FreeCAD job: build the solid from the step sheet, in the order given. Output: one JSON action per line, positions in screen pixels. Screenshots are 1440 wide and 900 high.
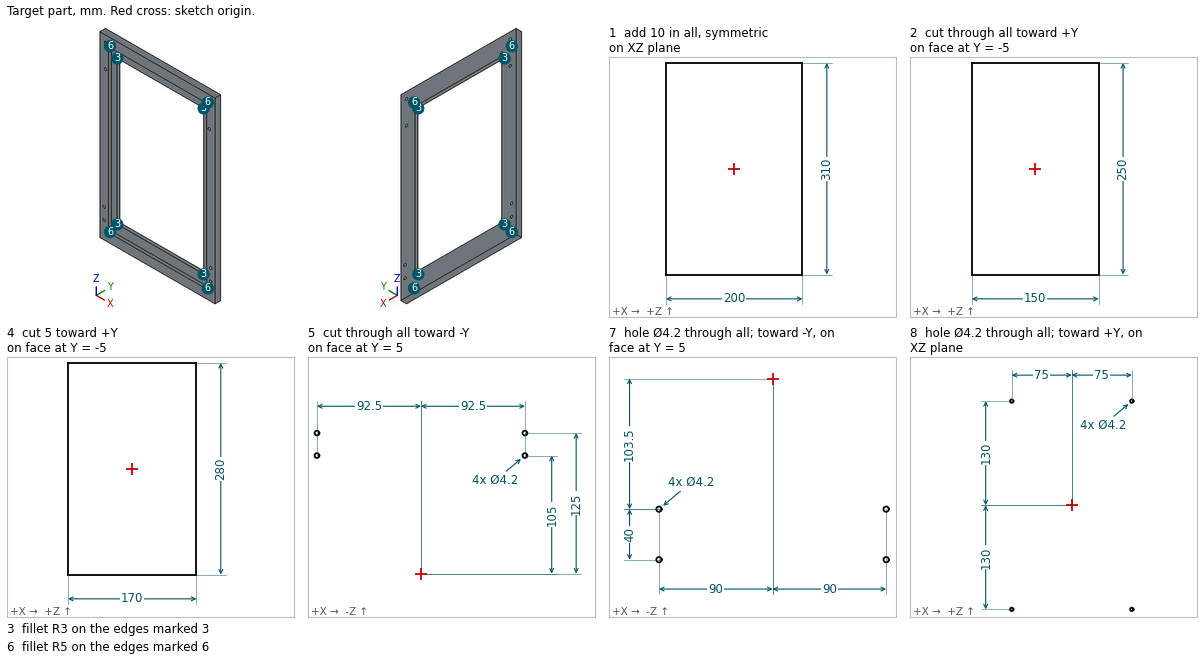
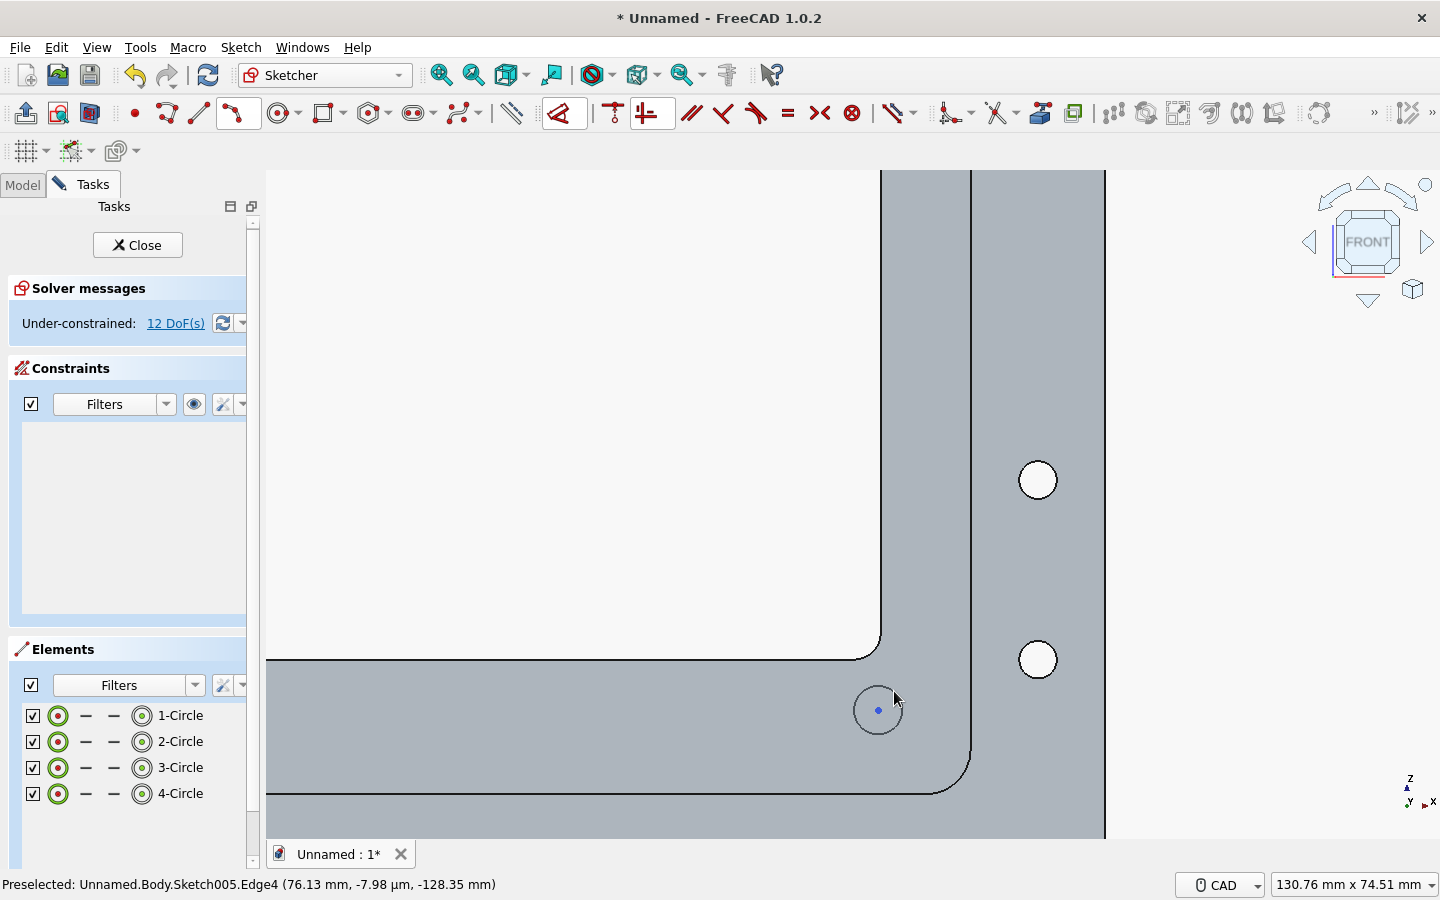
{"action": "scroll", "coordinate": [899, 696], "scroll_direction": "down", "scroll_amount": 9}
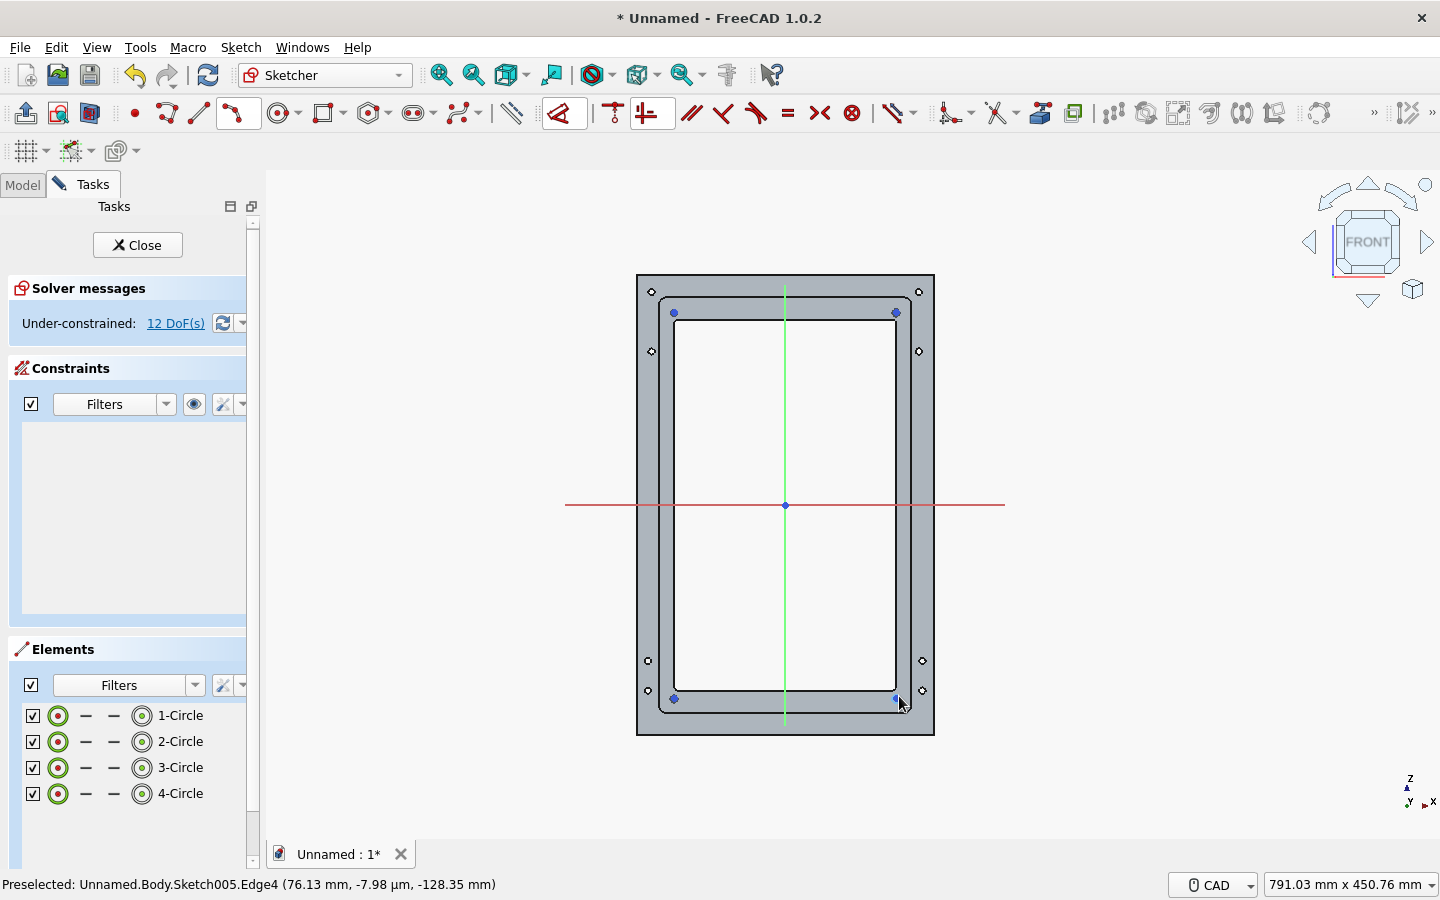
{"action": "scroll", "coordinate": [676, 311], "scroll_direction": "up", "scroll_amount": 8}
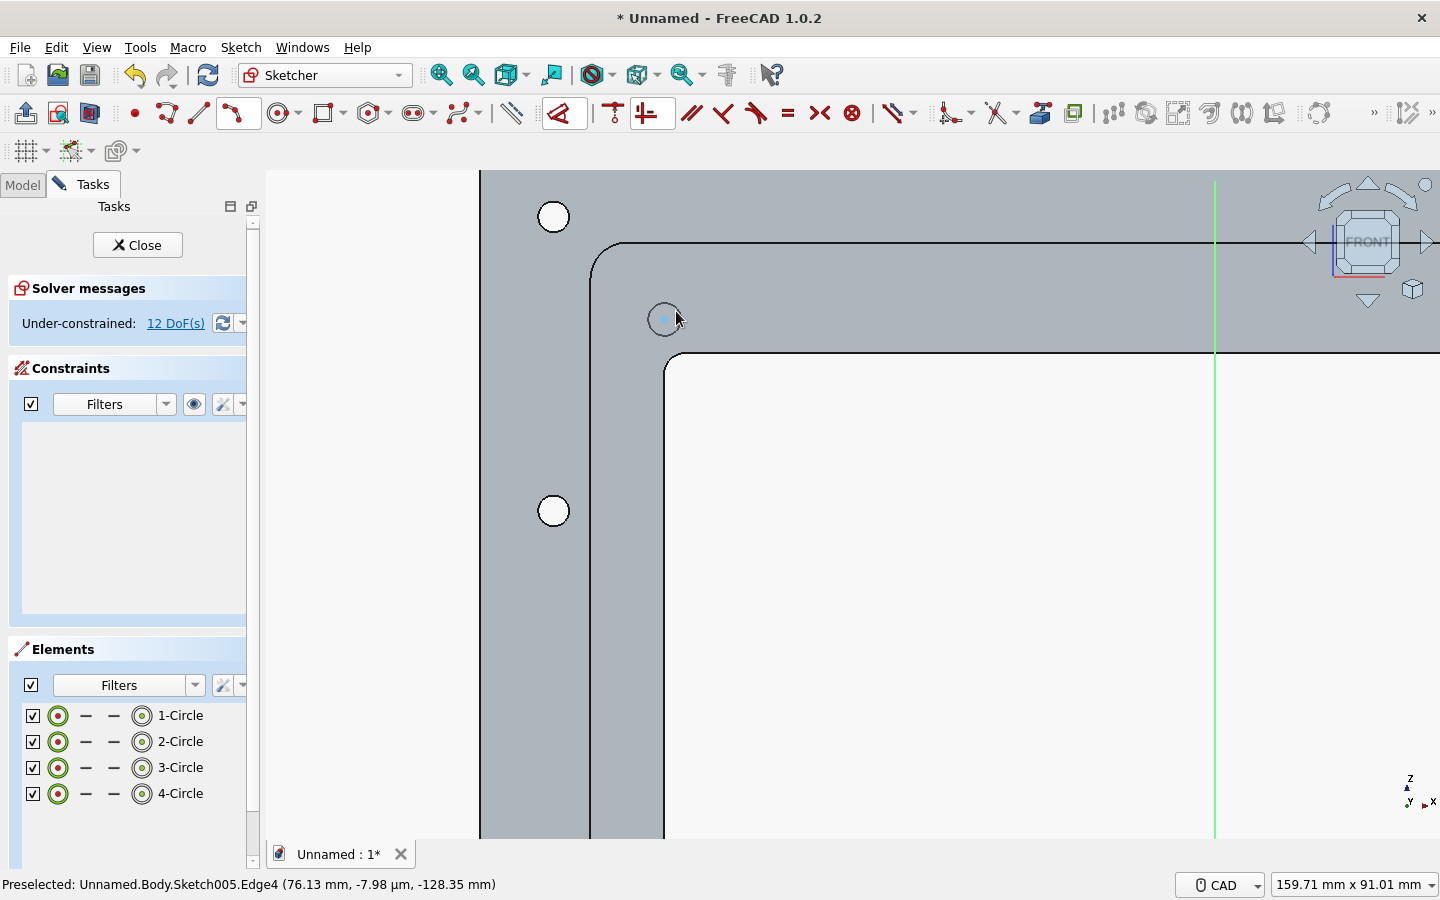
{"action": "left_click", "coordinate": [676, 308]}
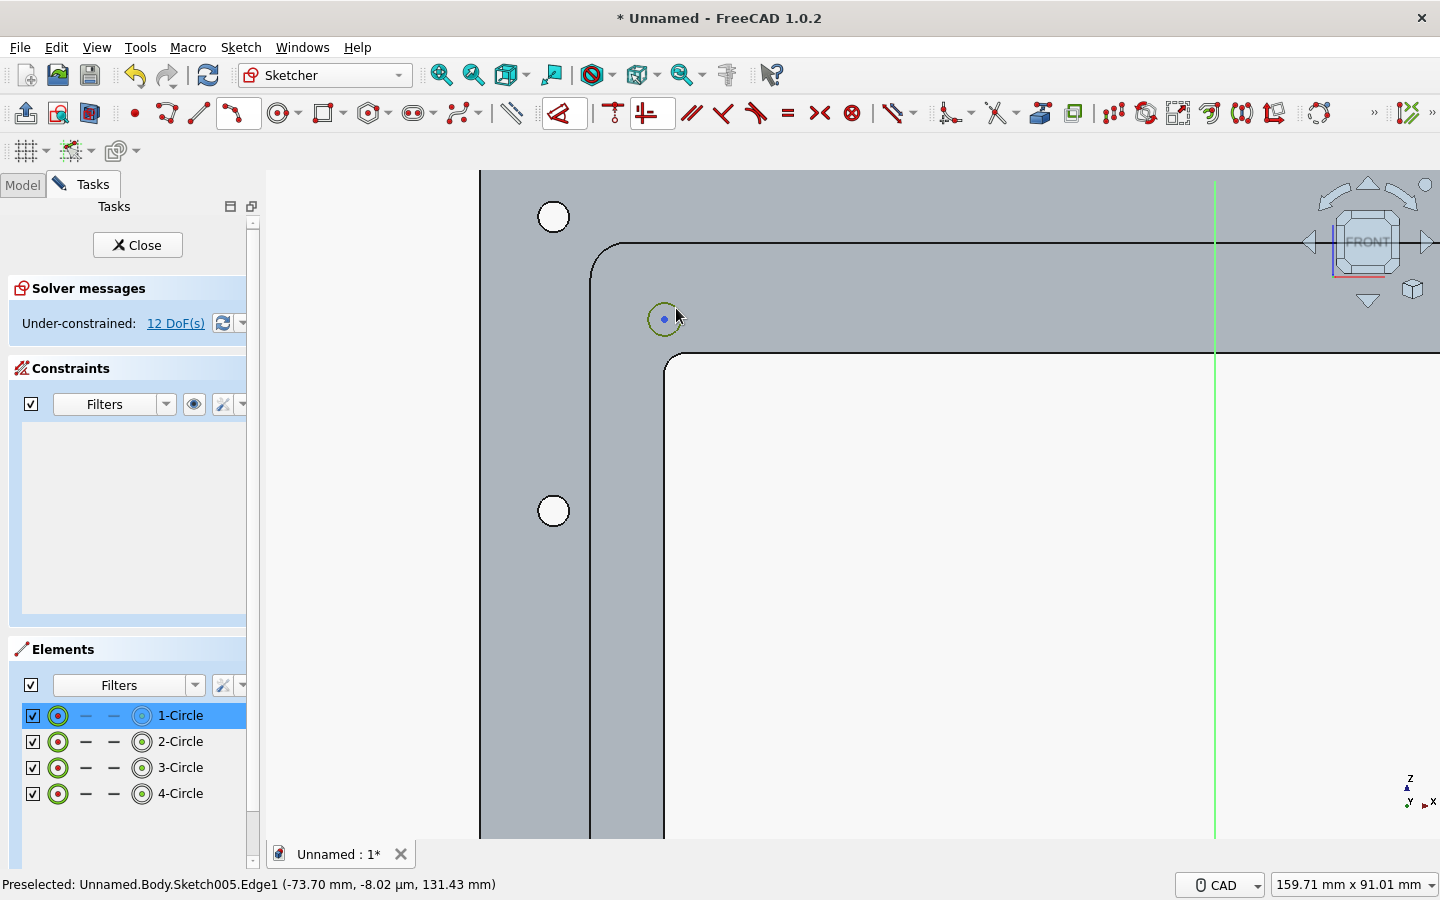
{"action": "scroll", "coordinate": [676, 310], "scroll_direction": "down", "scroll_amount": 8}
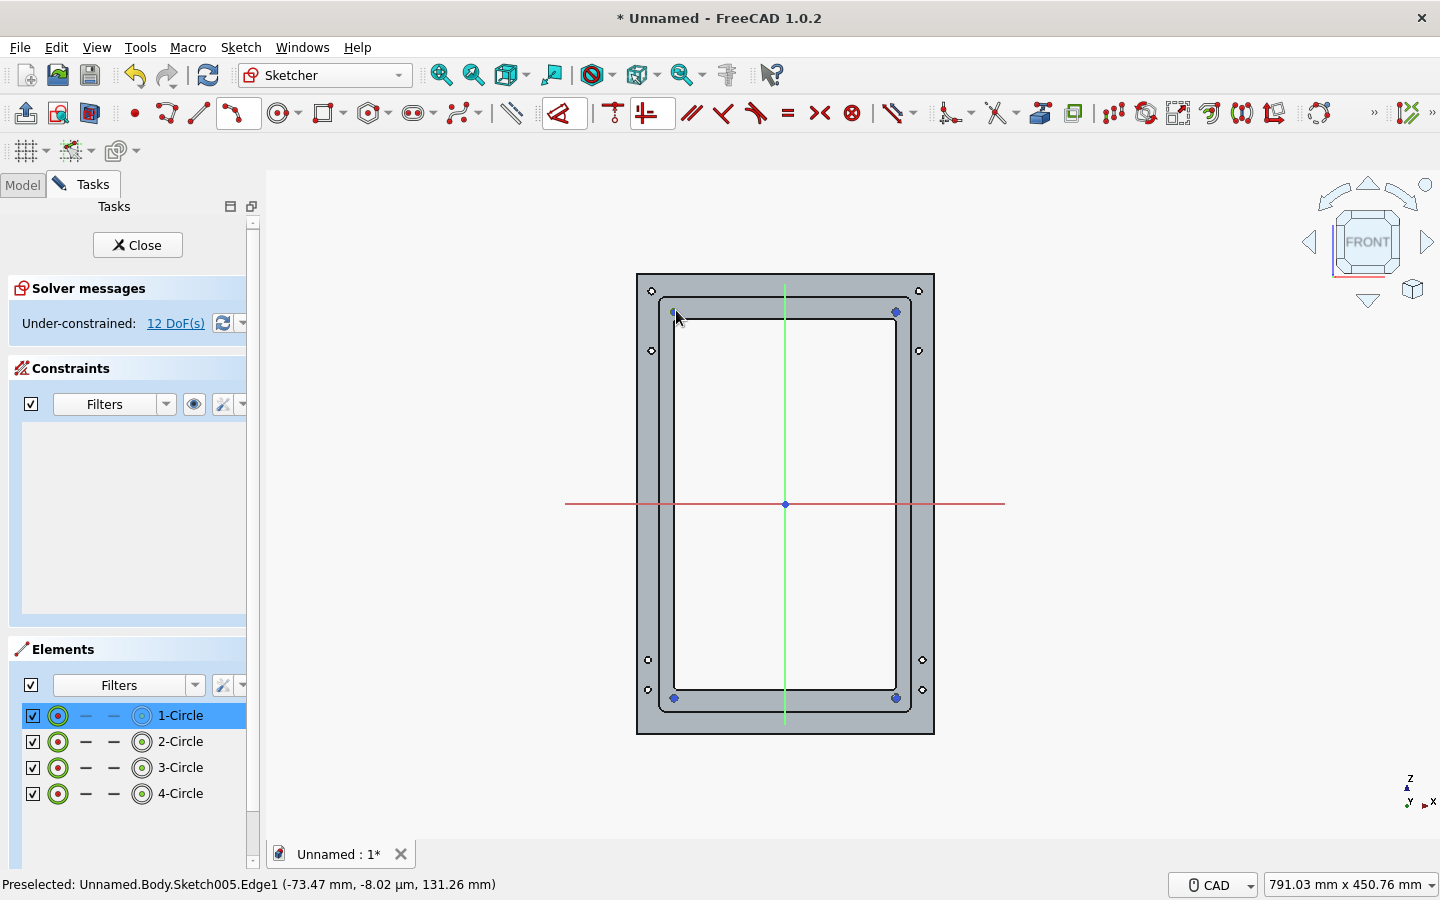
{"action": "scroll", "coordinate": [899, 309], "scroll_direction": "up", "scroll_amount": 7}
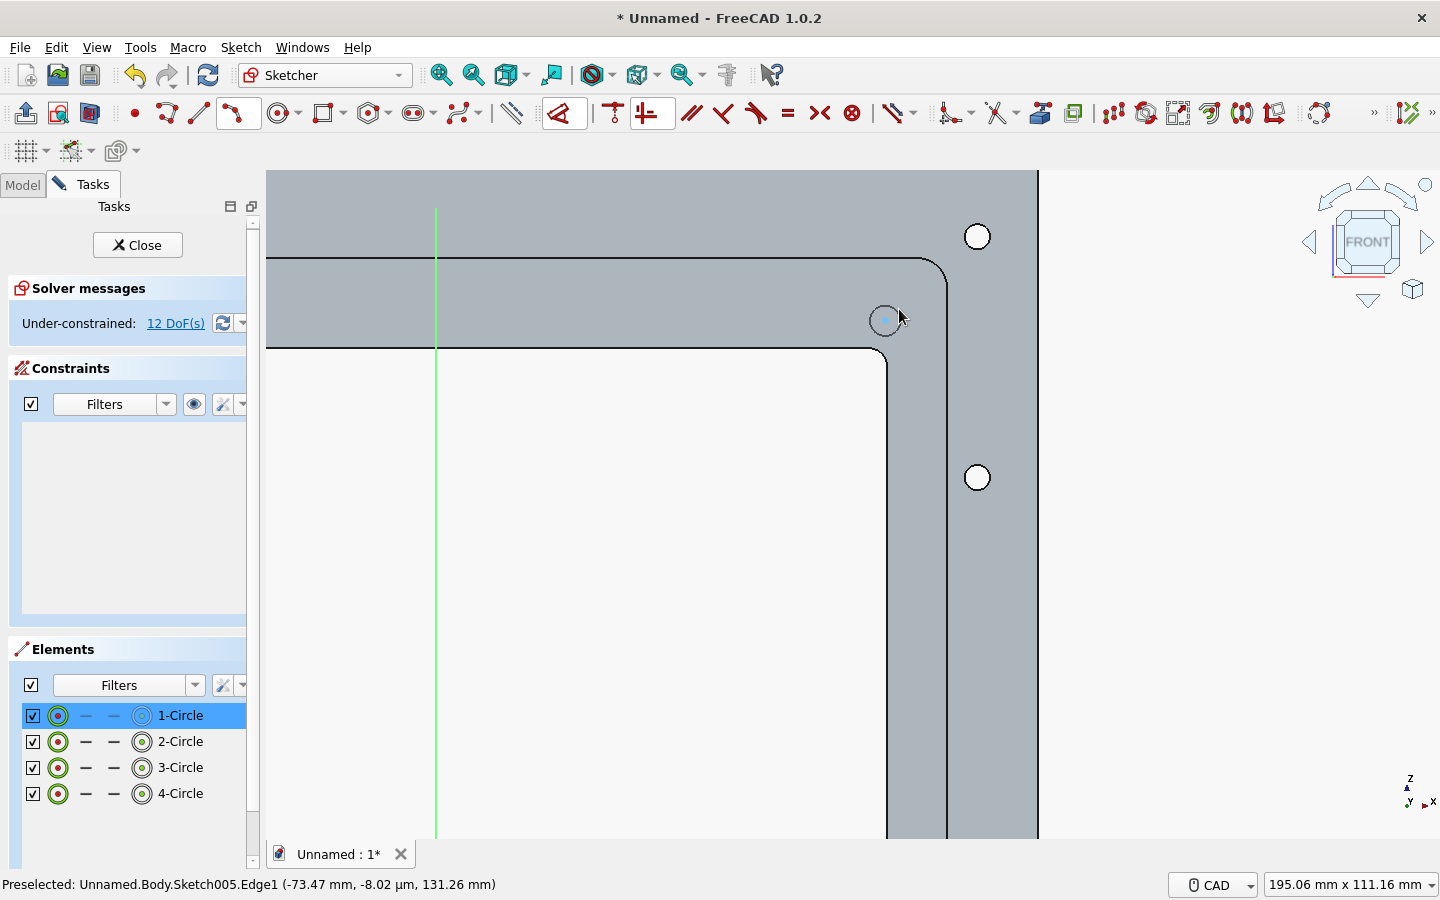
{"action": "left_click", "coordinate": [896, 310]}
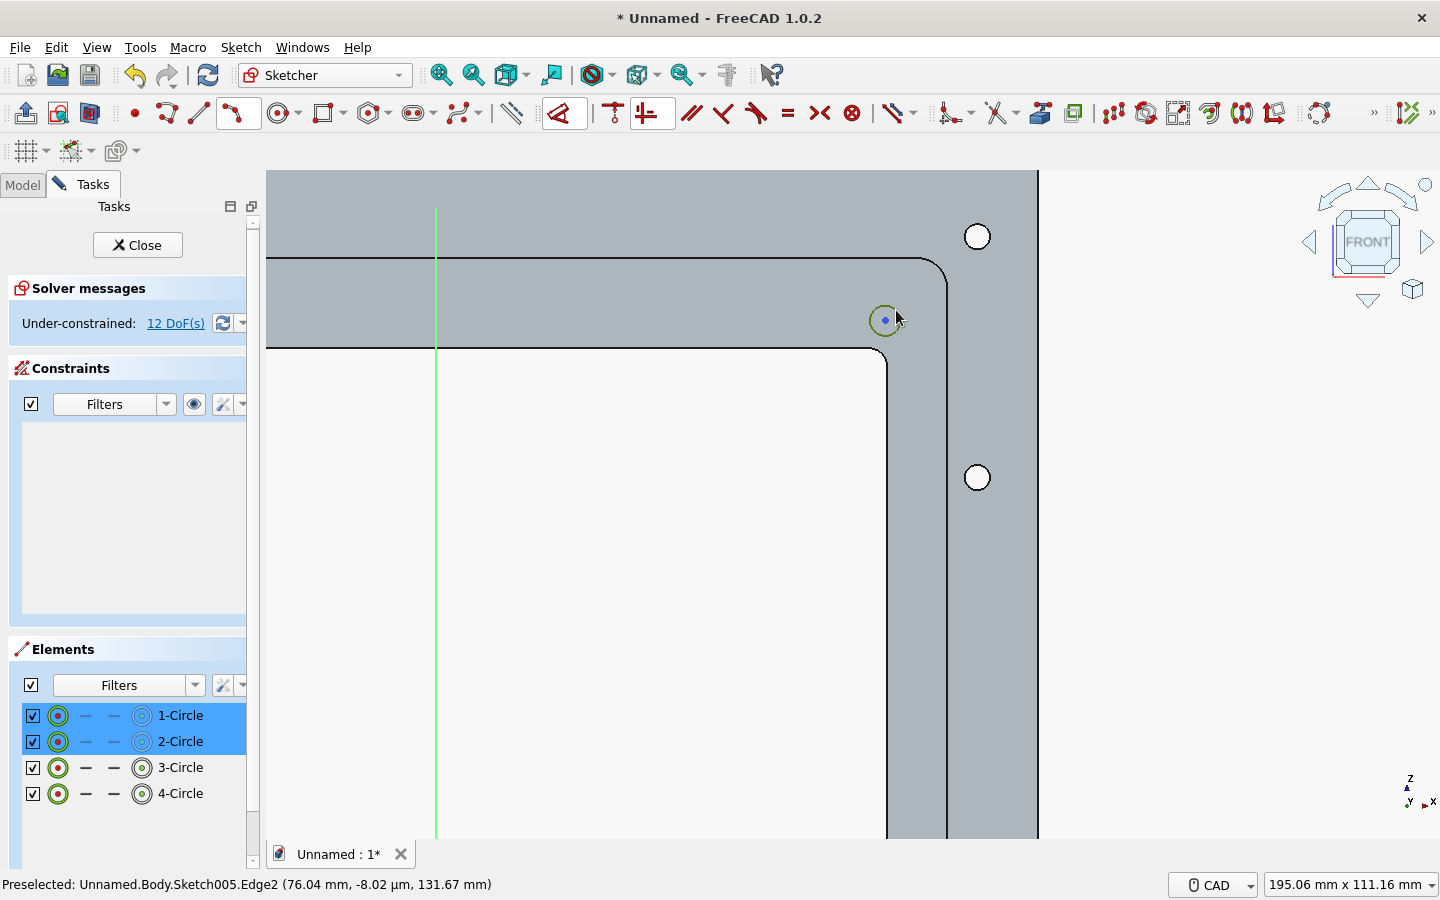
{"action": "scroll", "coordinate": [899, 309], "scroll_direction": "down", "scroll_amount": 7}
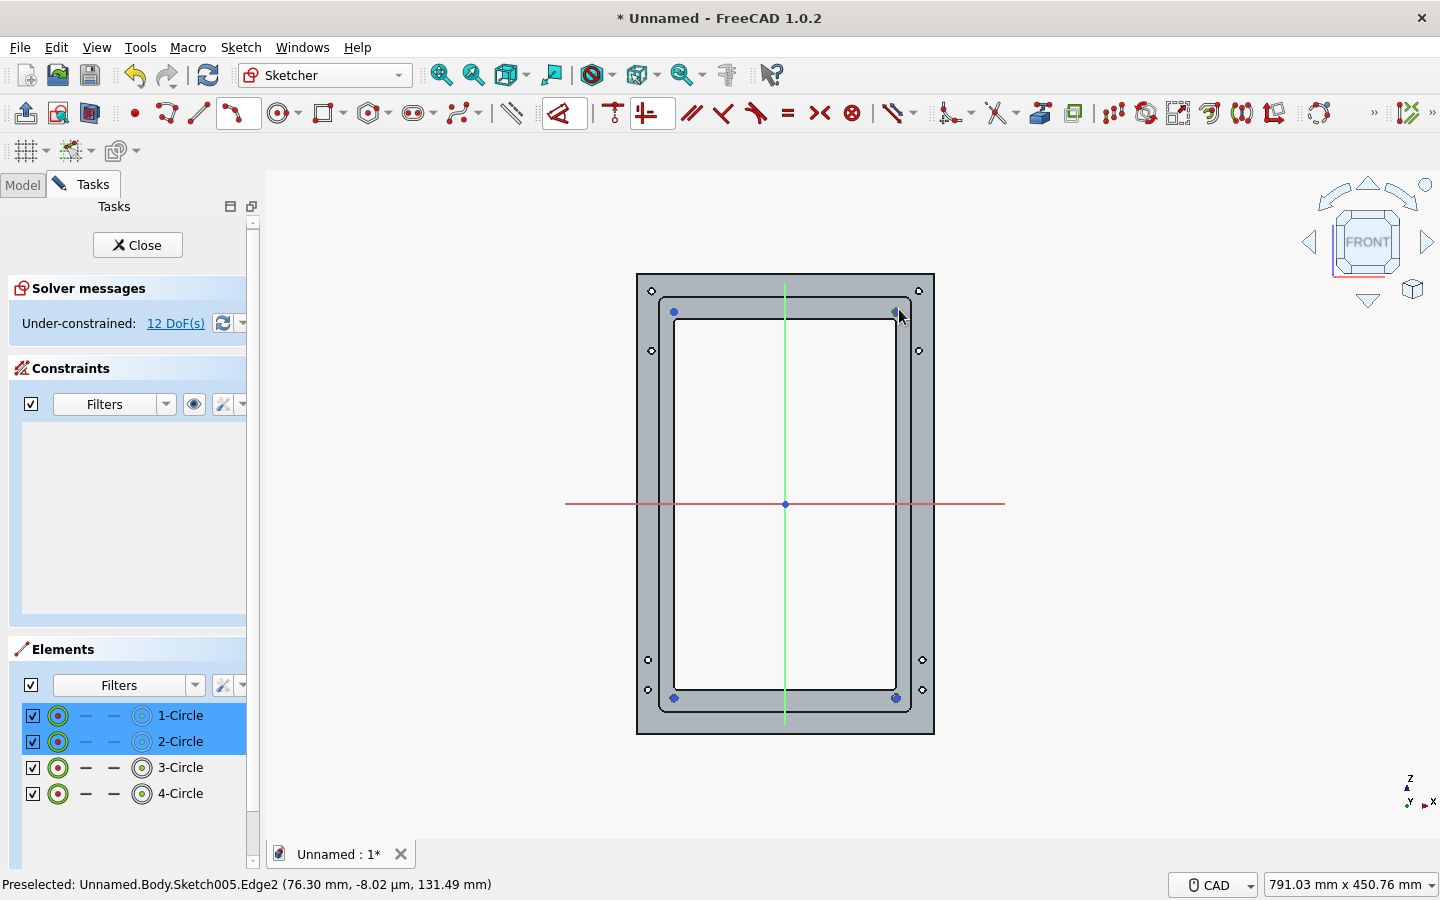
{"action": "scroll", "coordinate": [677, 696], "scroll_direction": "up", "scroll_amount": 7}